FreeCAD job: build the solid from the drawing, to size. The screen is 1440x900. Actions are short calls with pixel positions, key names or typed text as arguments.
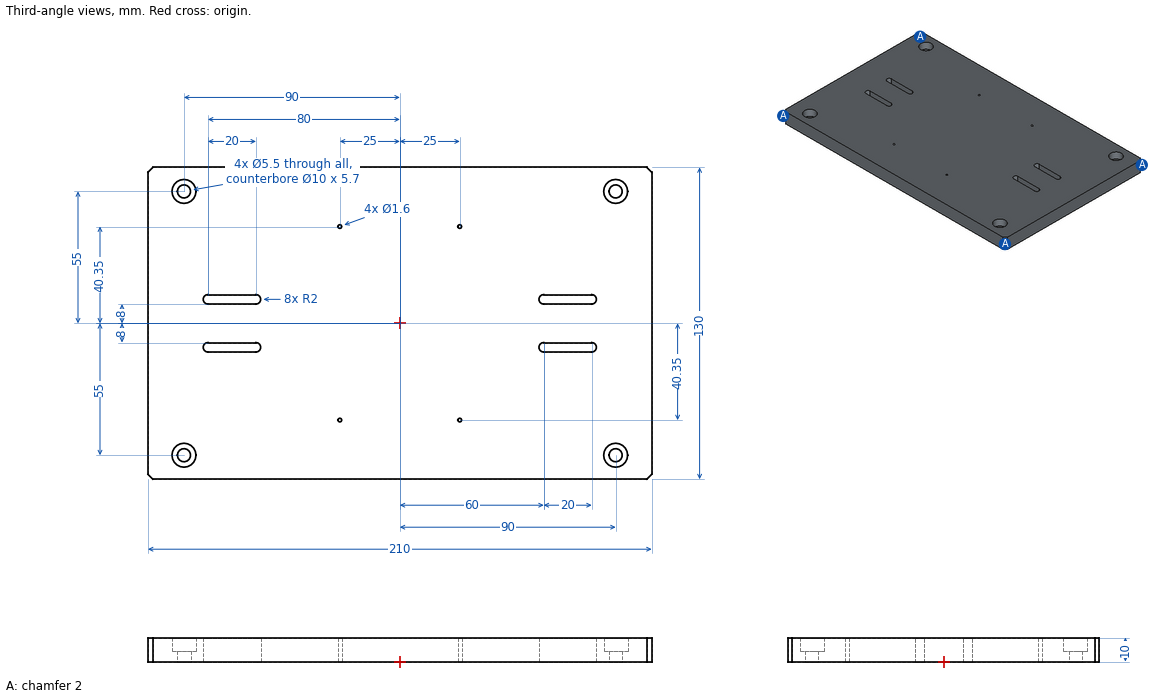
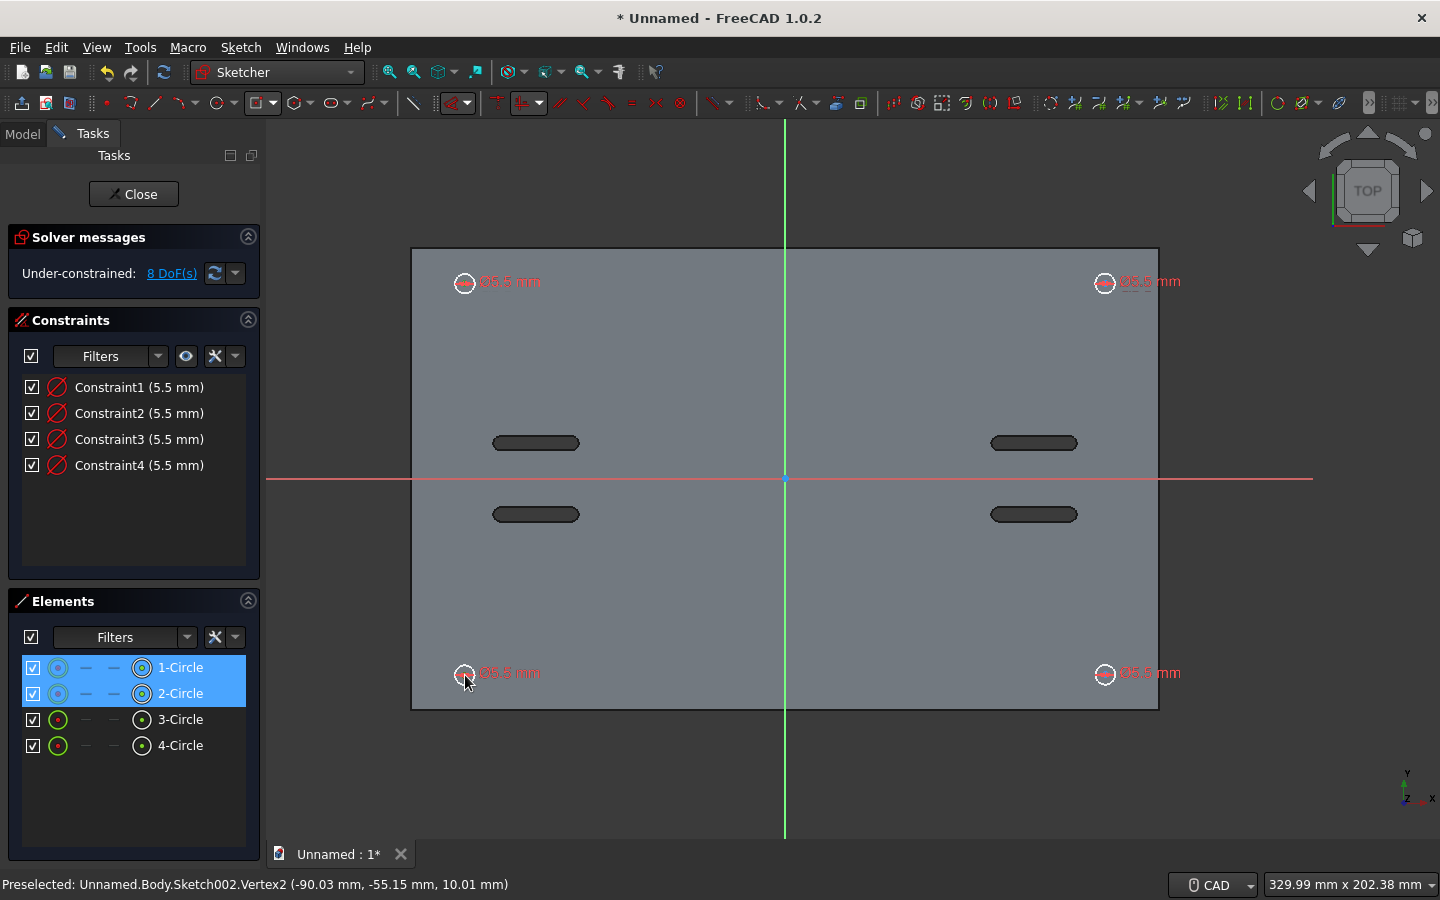
key(v)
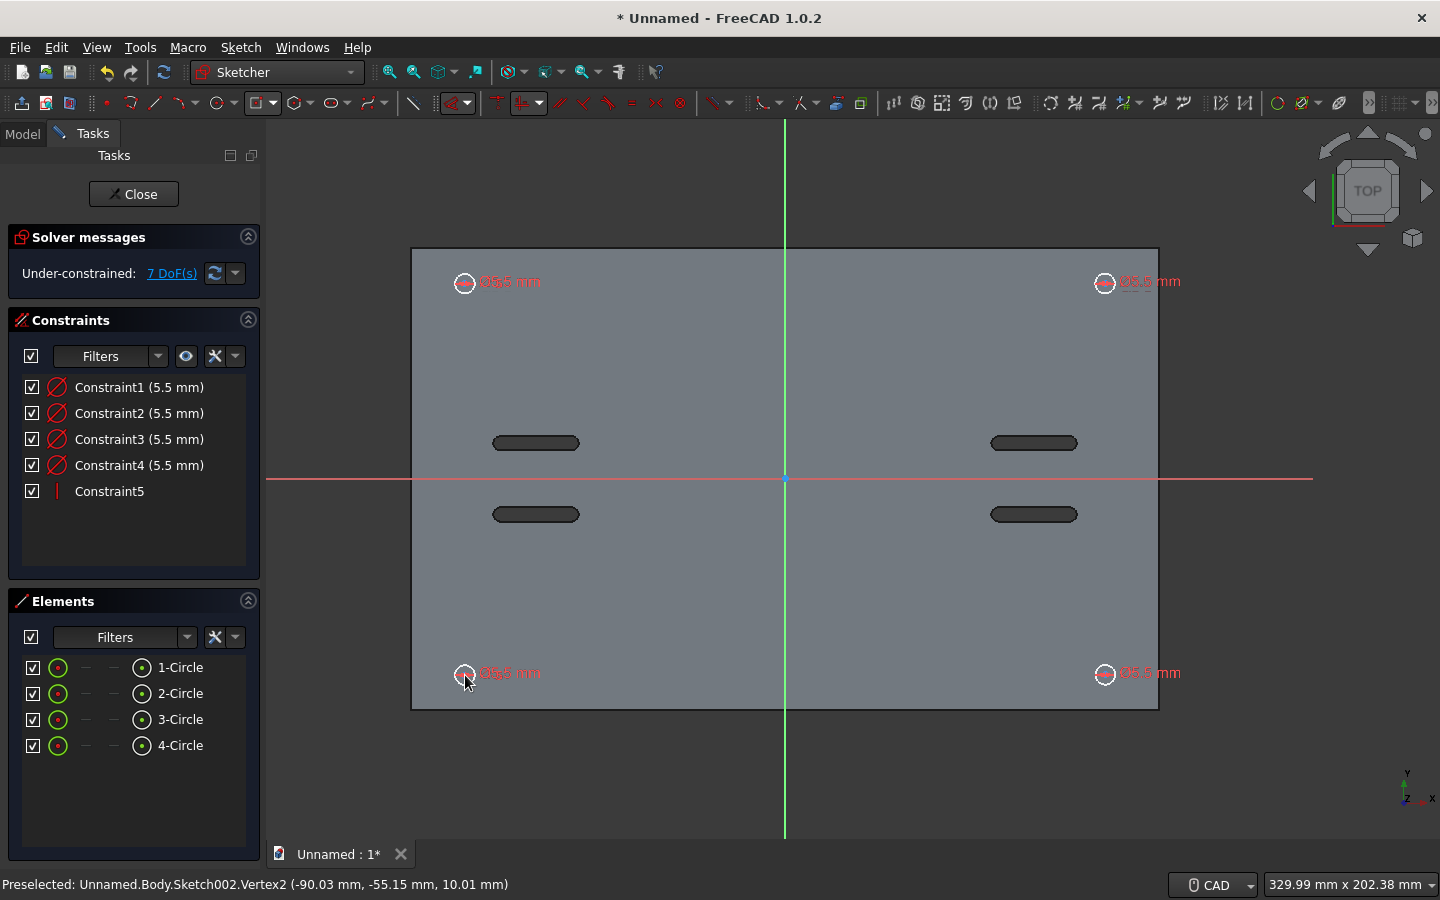
click(465, 675)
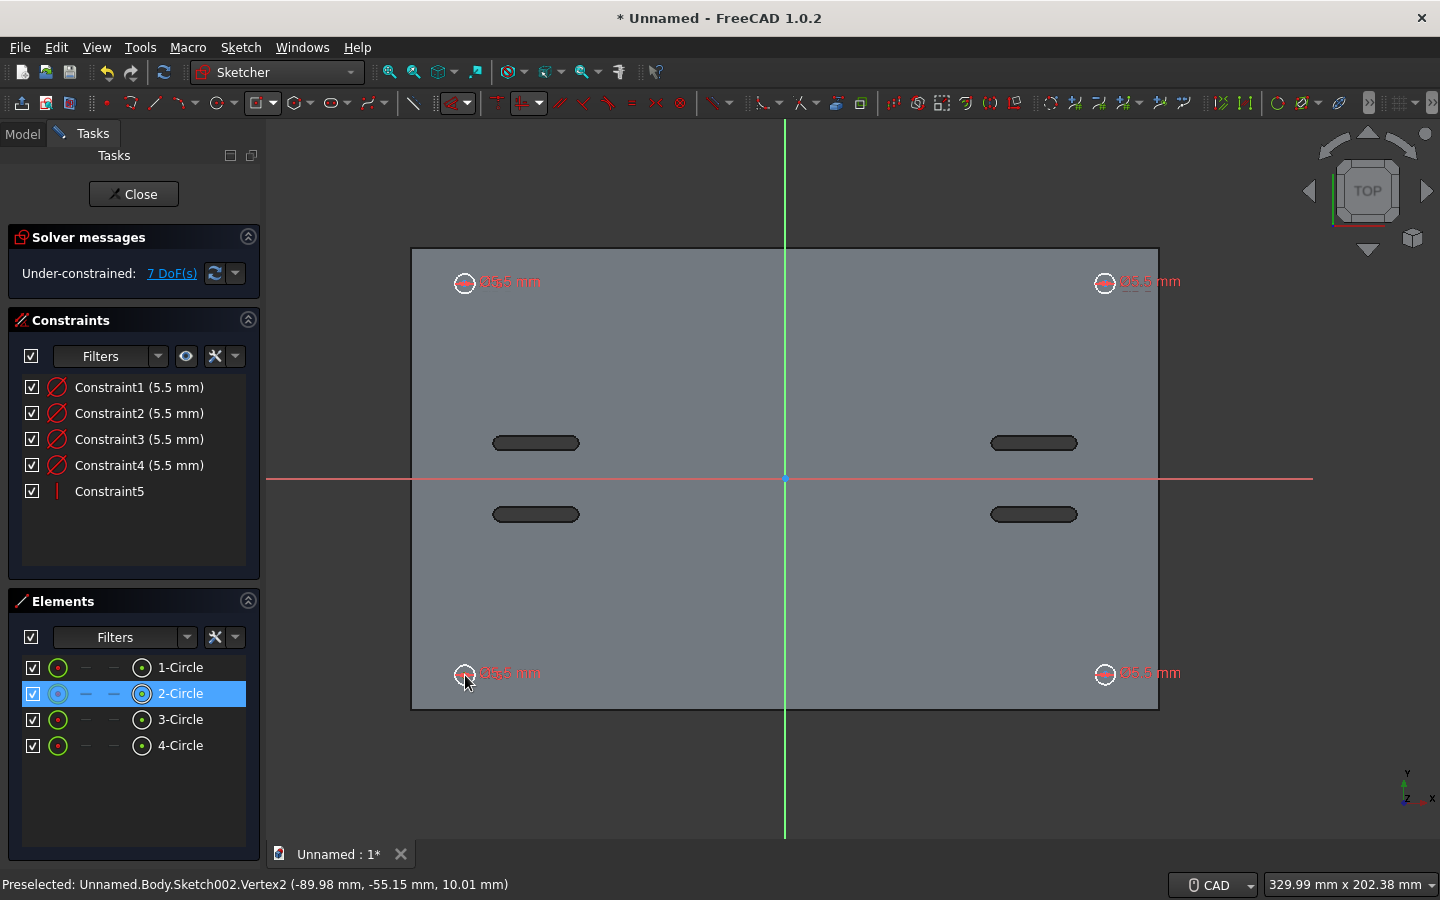
click(1105, 675)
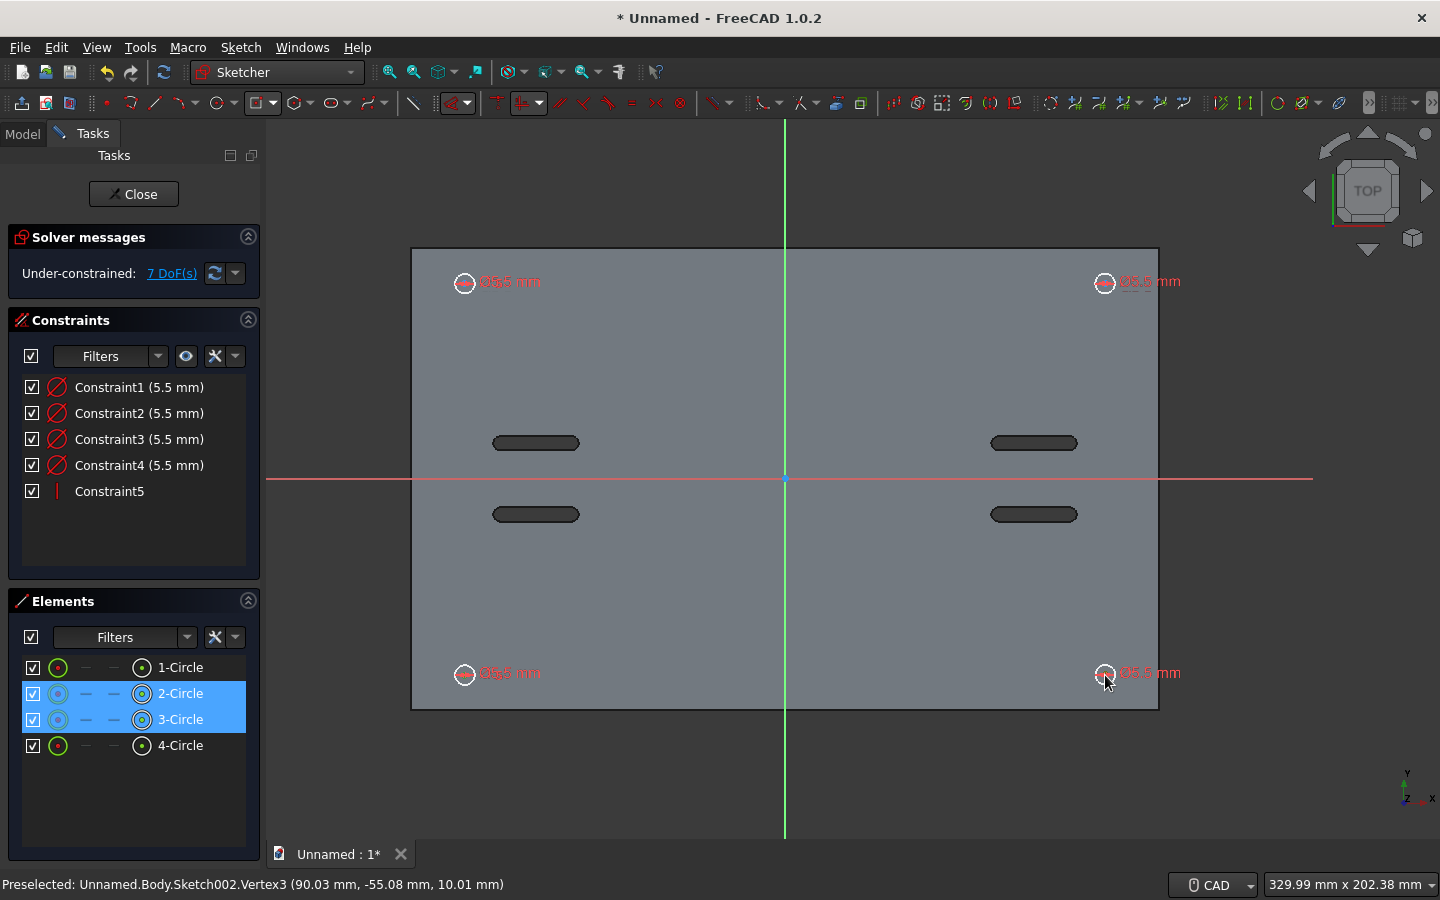
key(h)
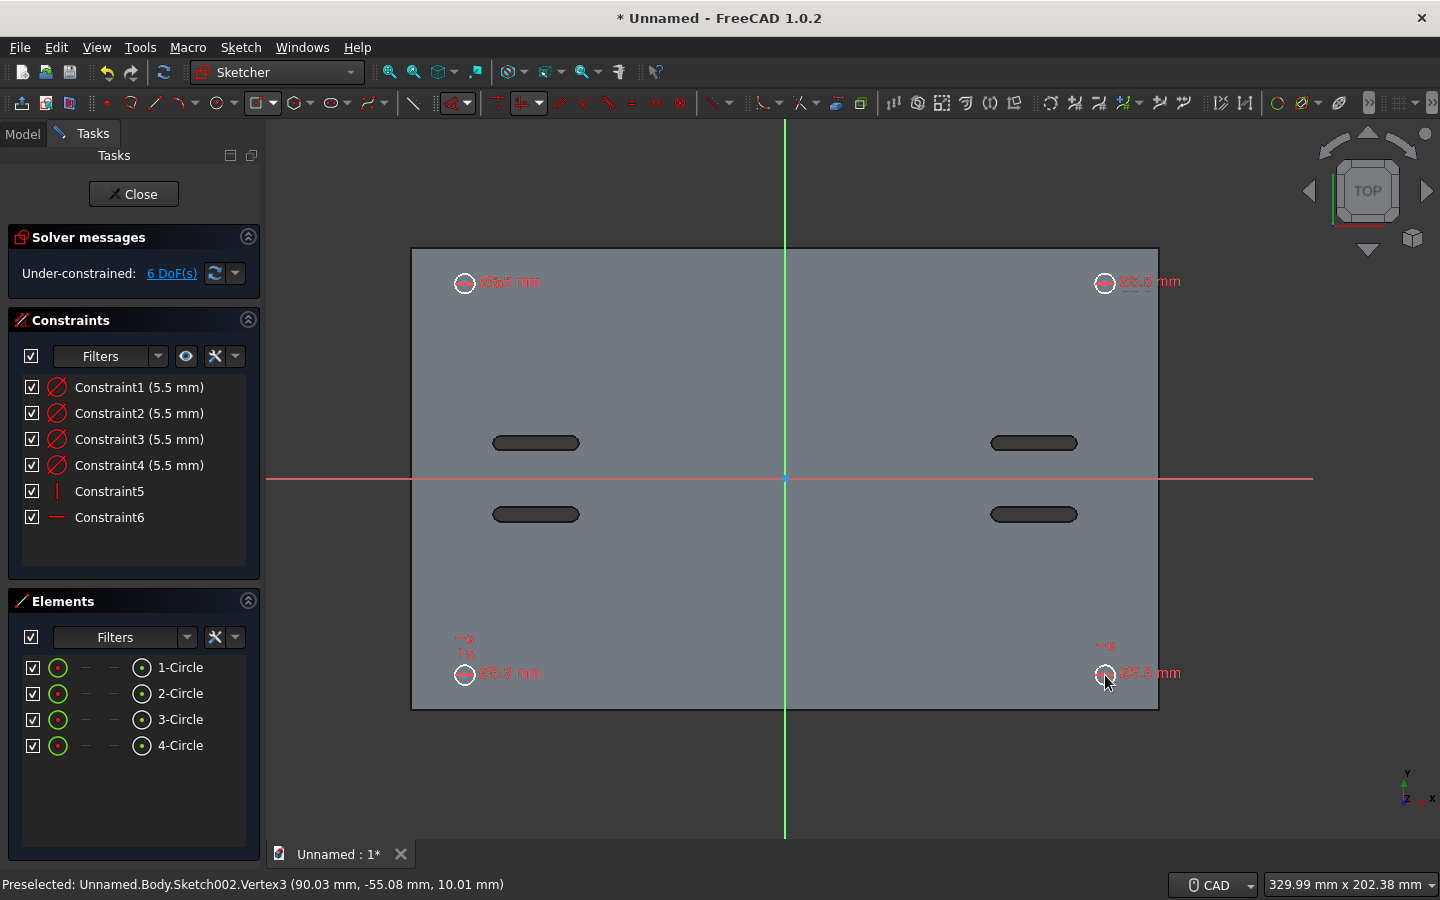
click(1105, 675)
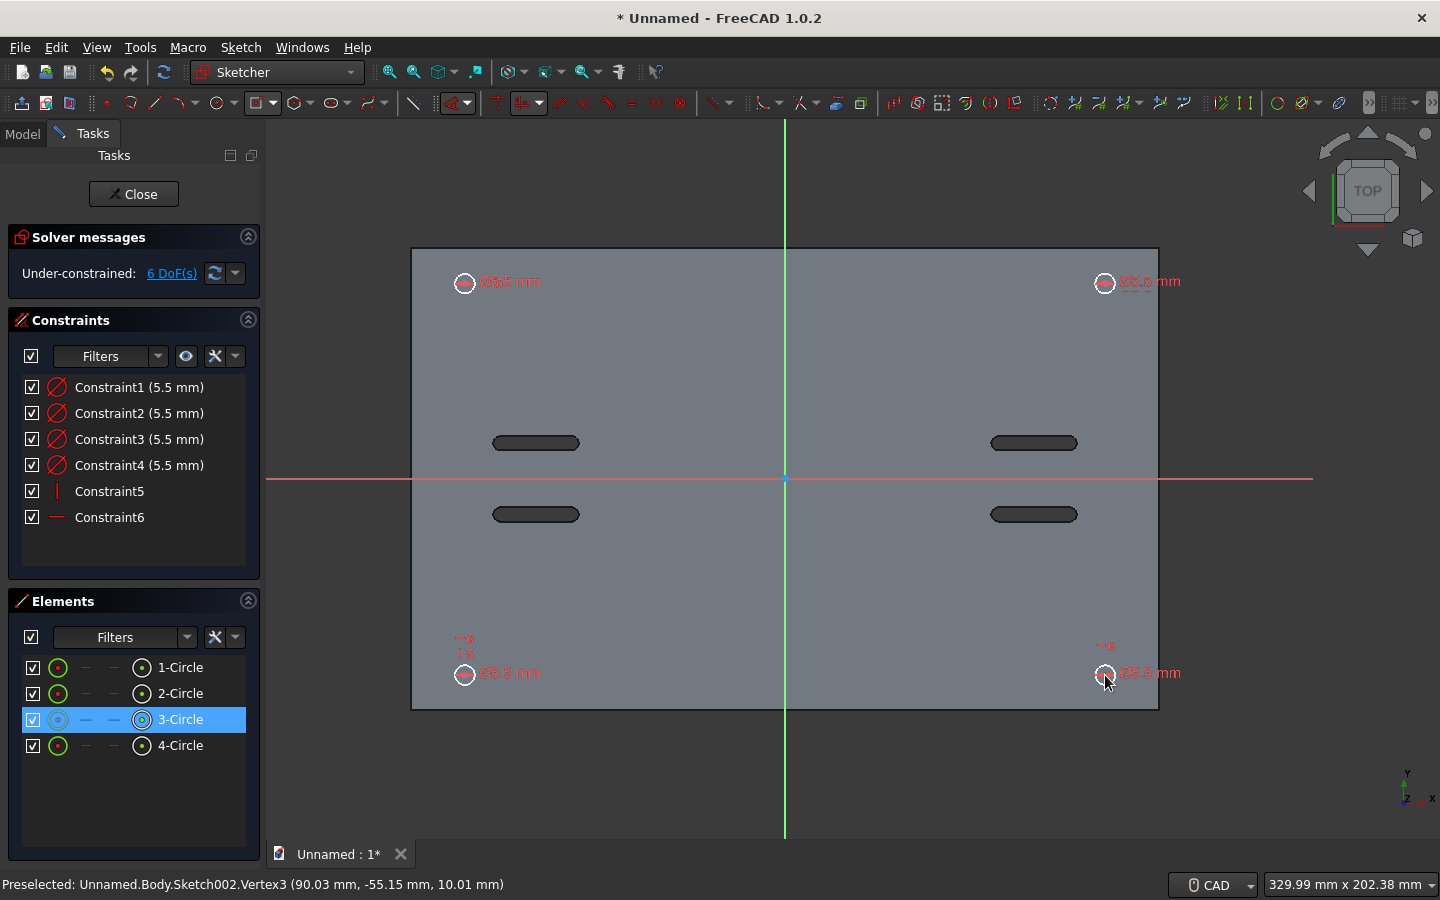
click(1105, 284)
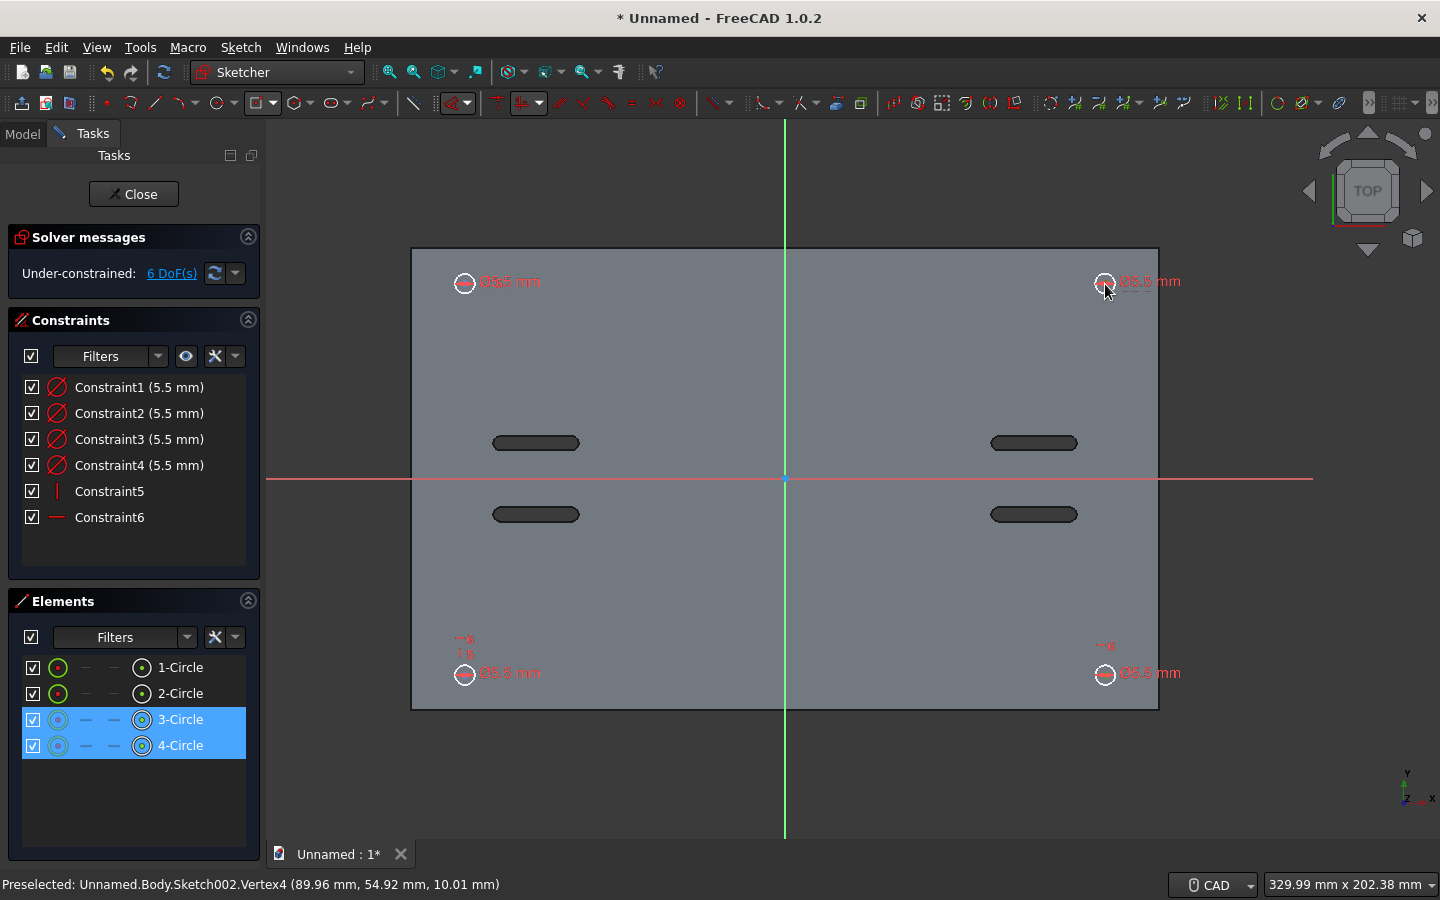
click(542, 104)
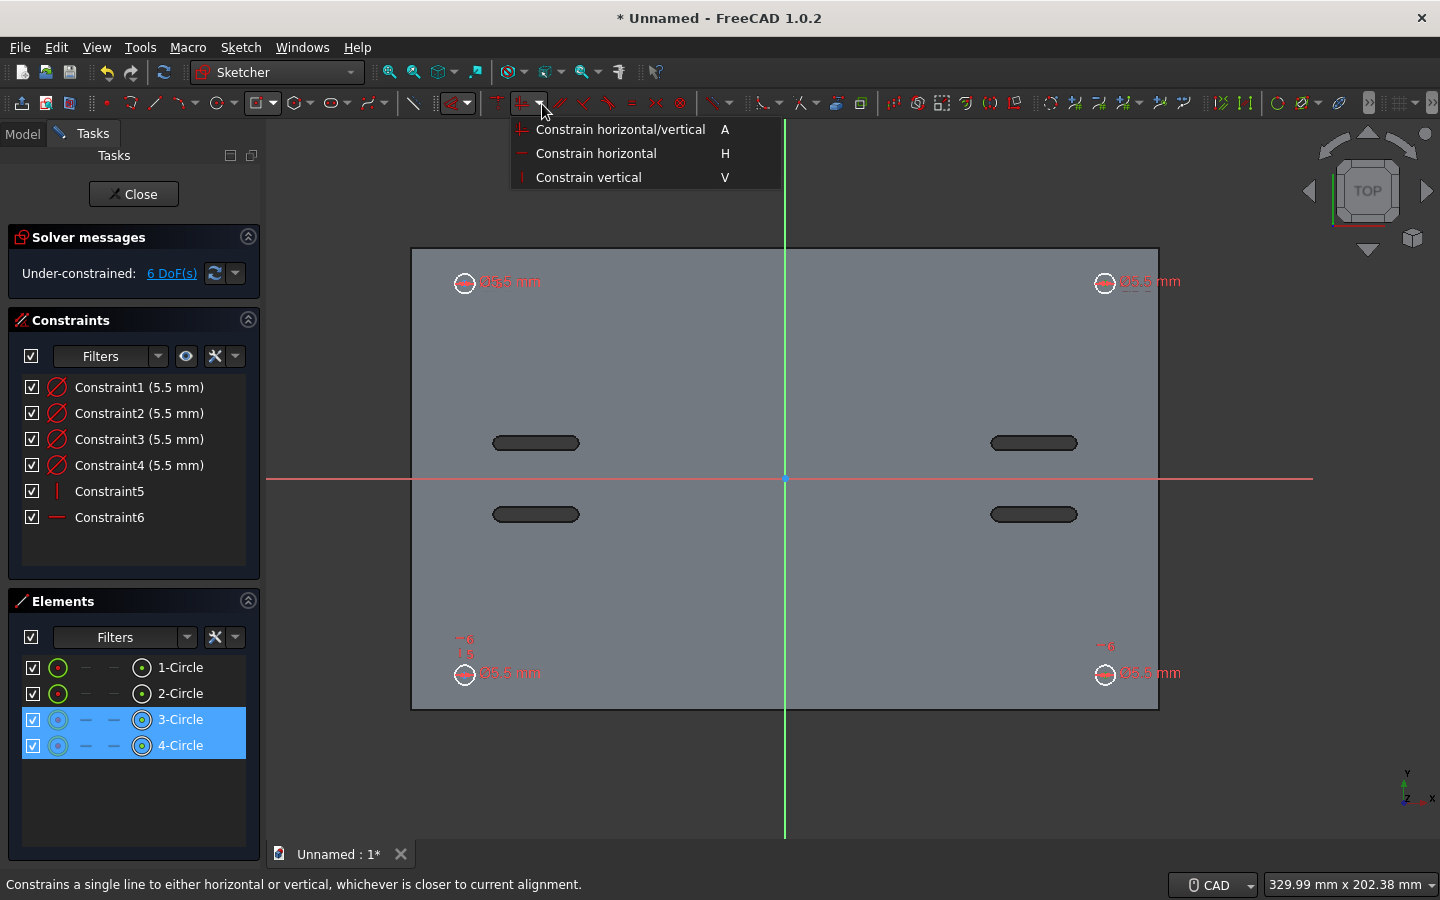
click(646, 177)